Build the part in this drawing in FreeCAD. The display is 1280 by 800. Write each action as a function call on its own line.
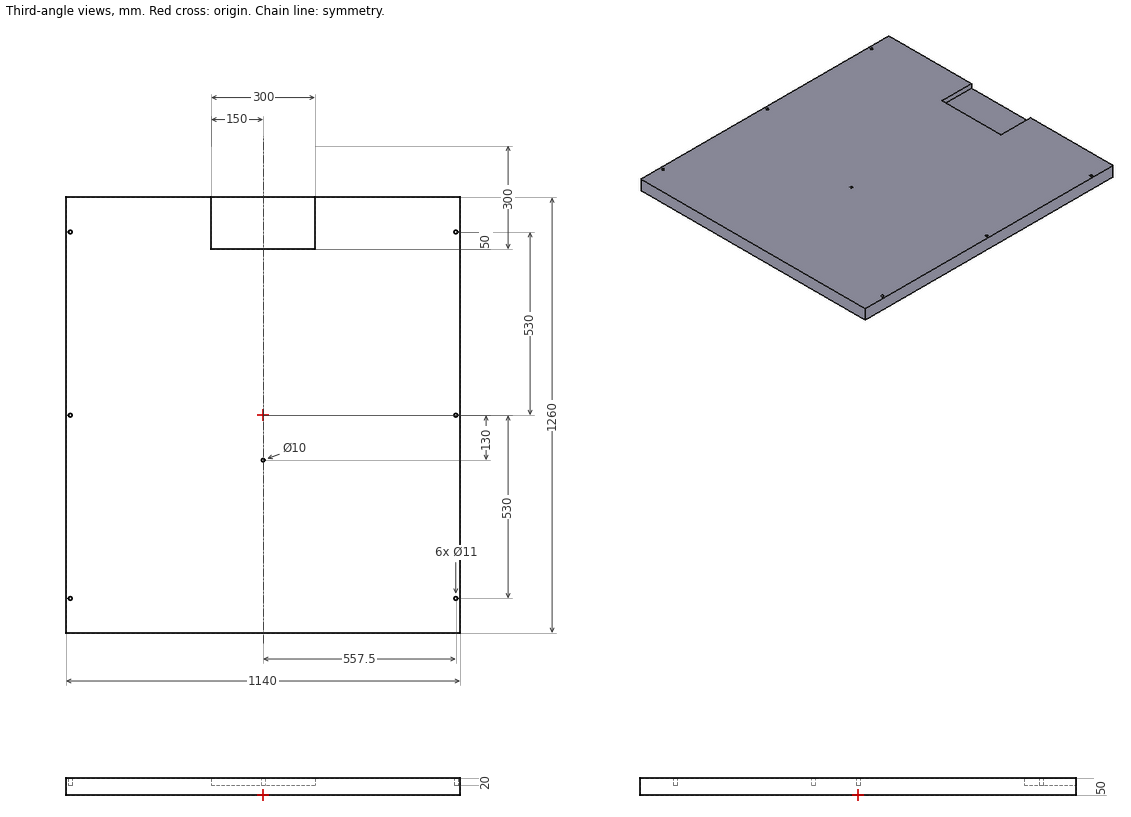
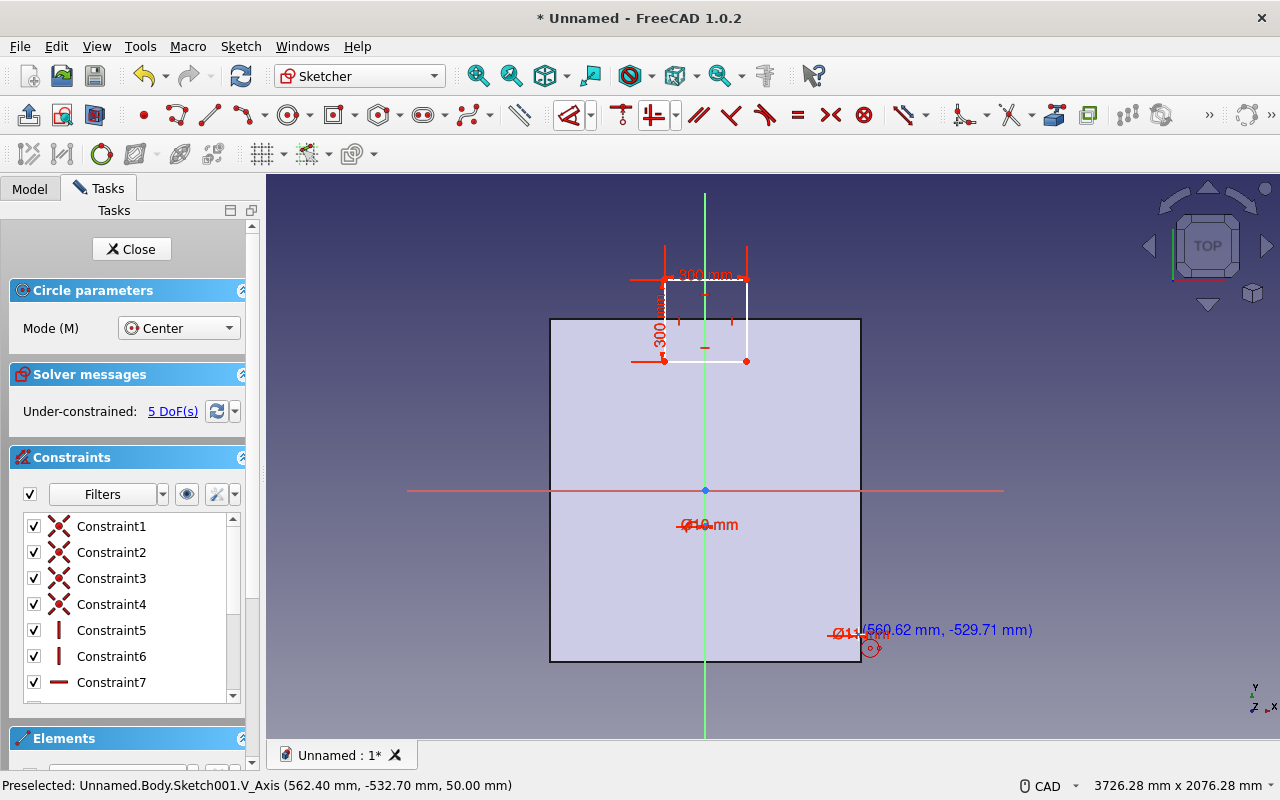
scroll(857, 491, up, 14)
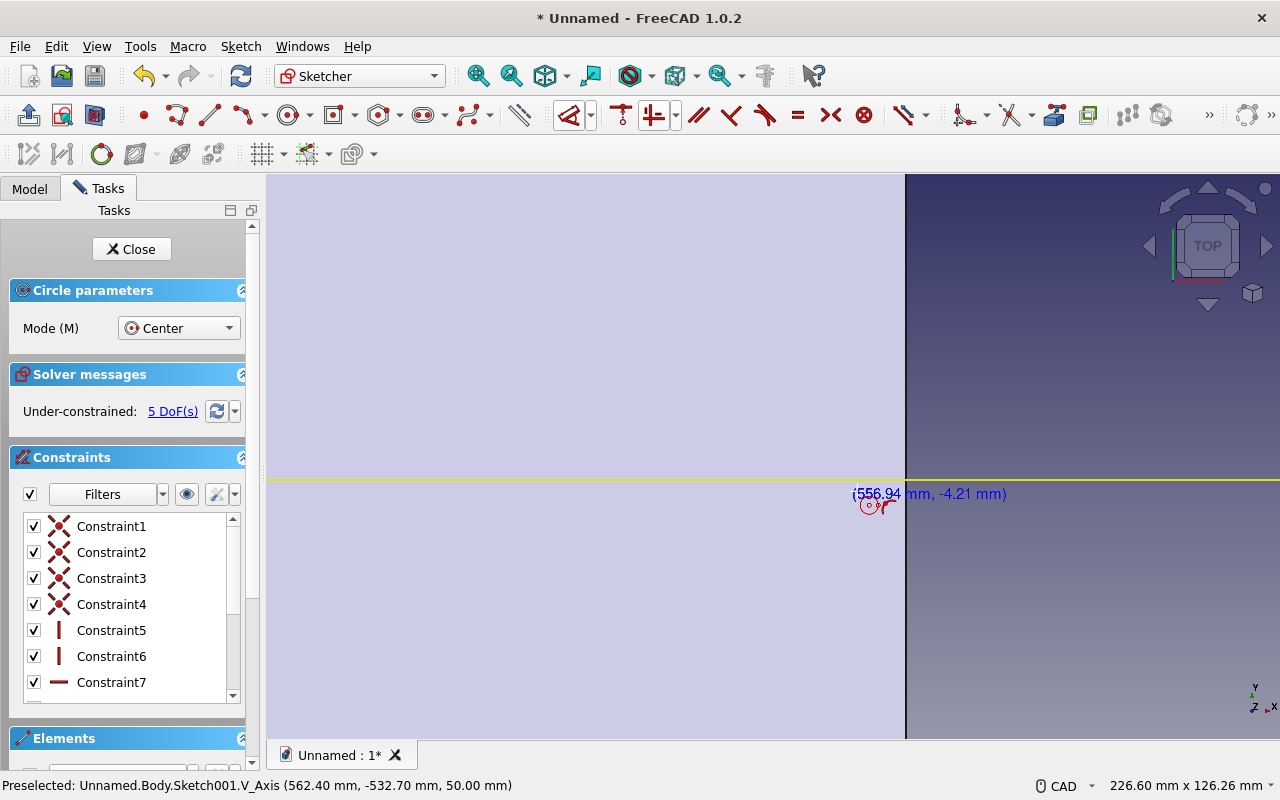
scroll(857, 490, down, 14)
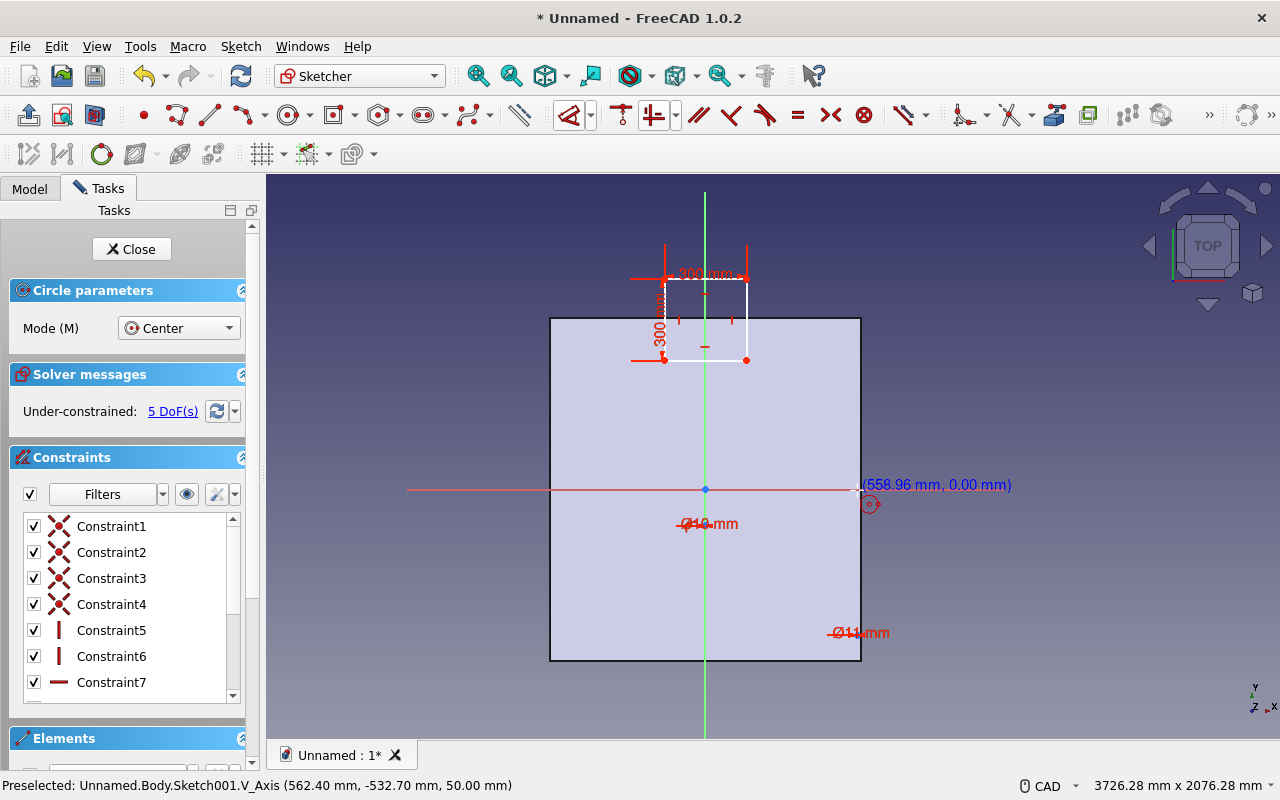
click(857, 490)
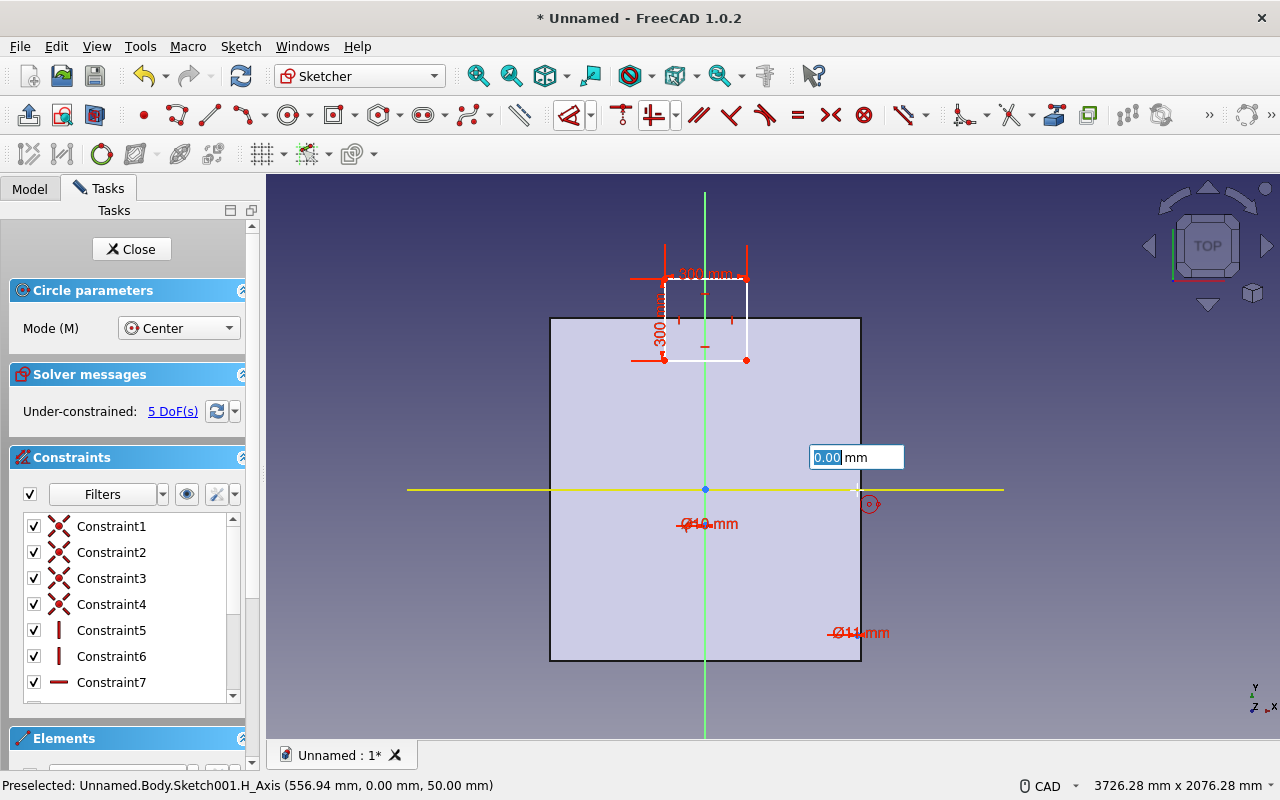
scroll(858, 489, up, 13)
move(846, 475)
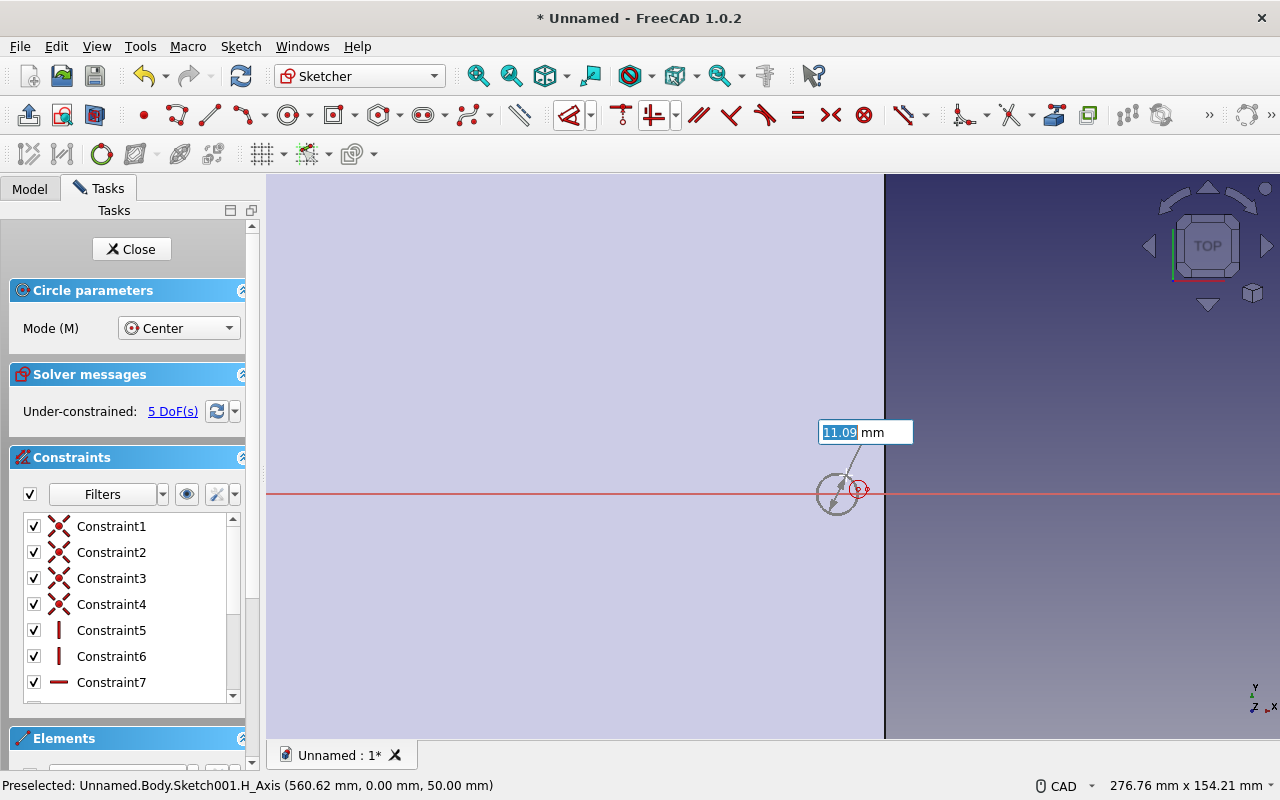
text(11)
key(Return)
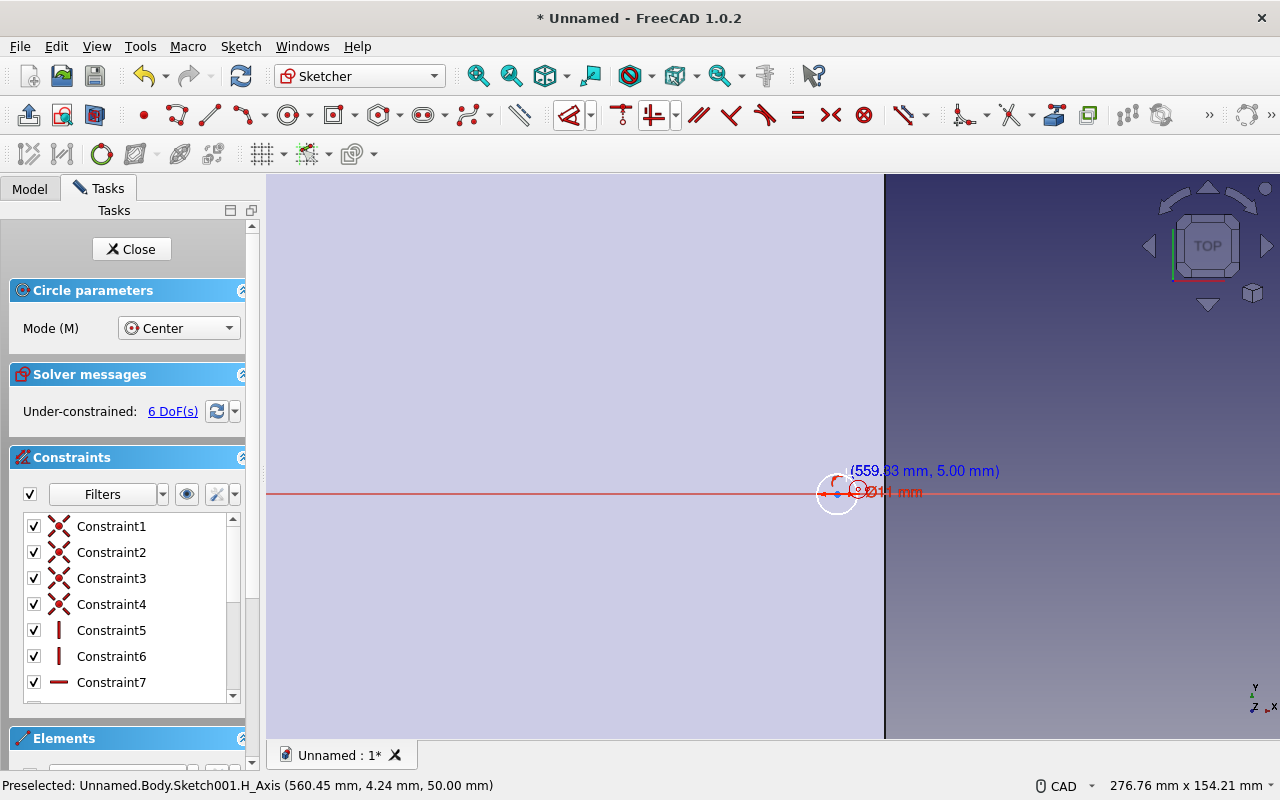
scroll(858, 489, down, 13)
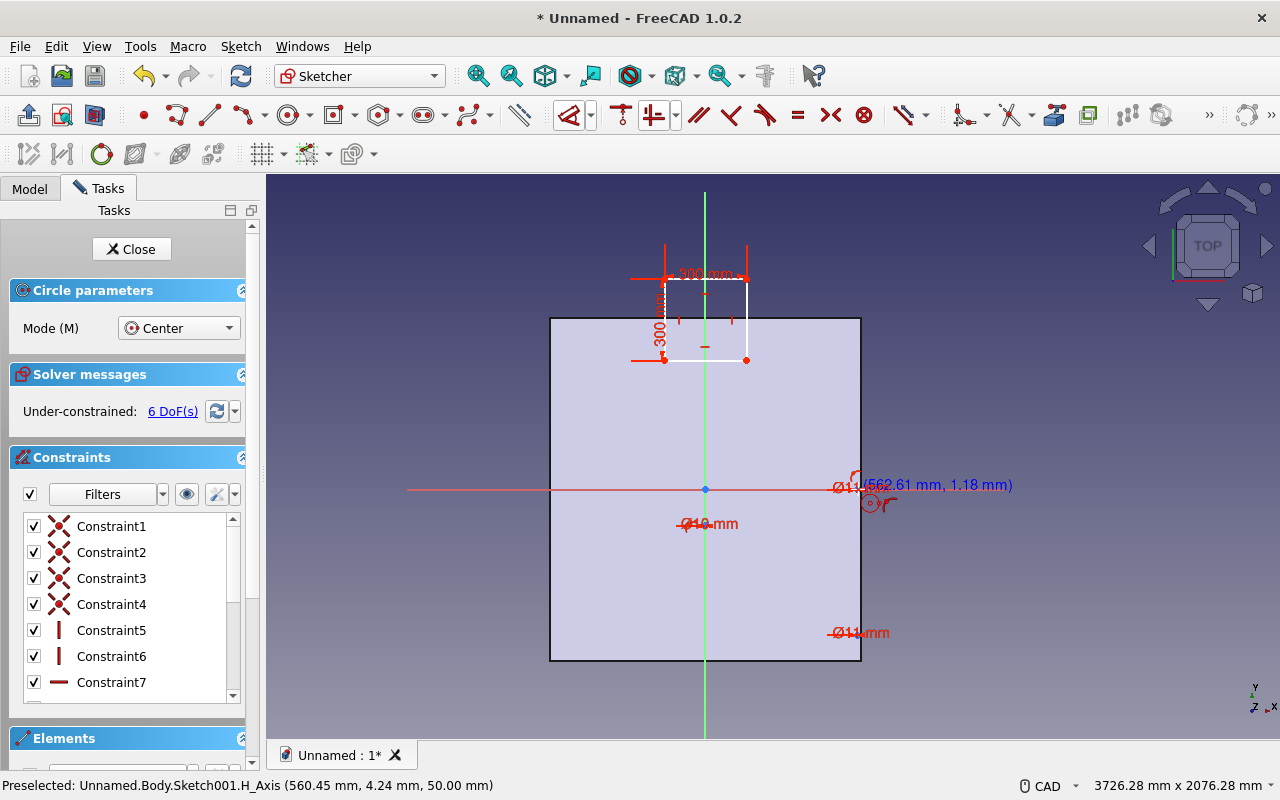
scroll(857, 346, up, 14)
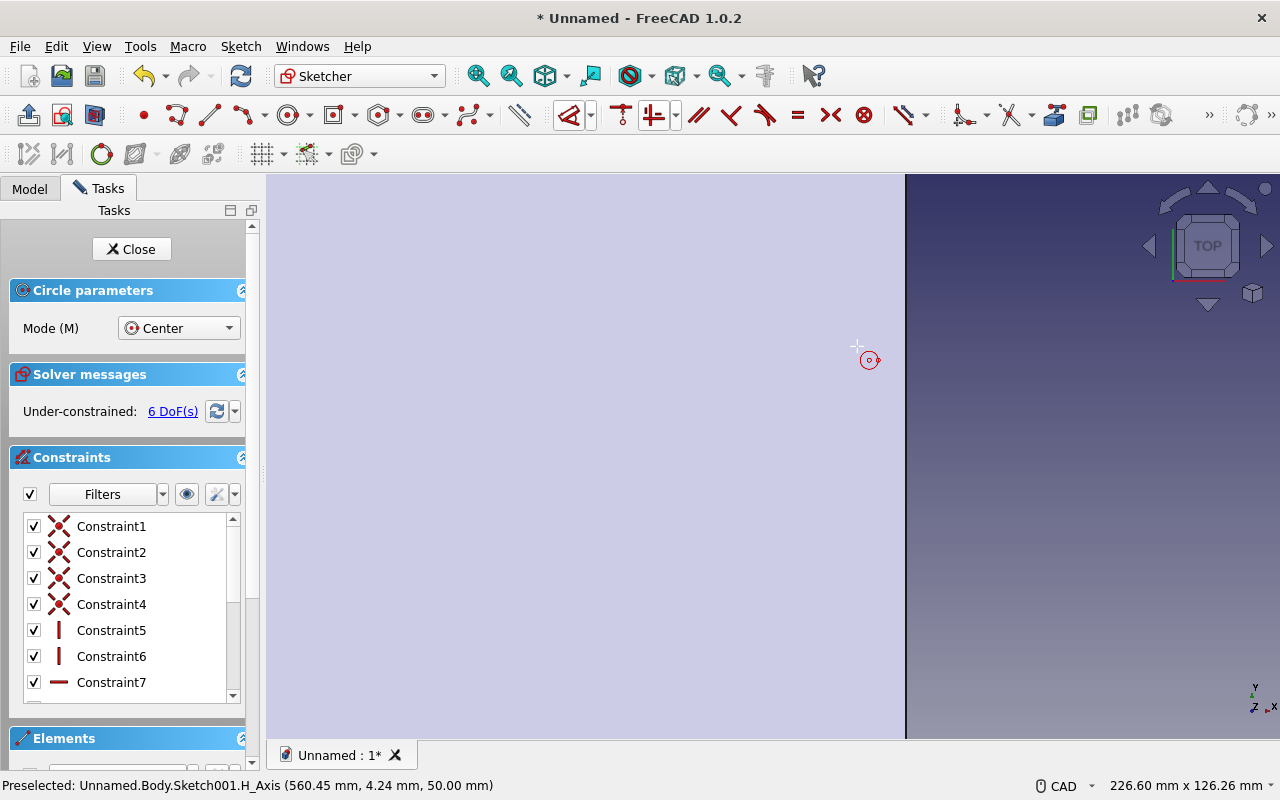
scroll(857, 346, down, 14)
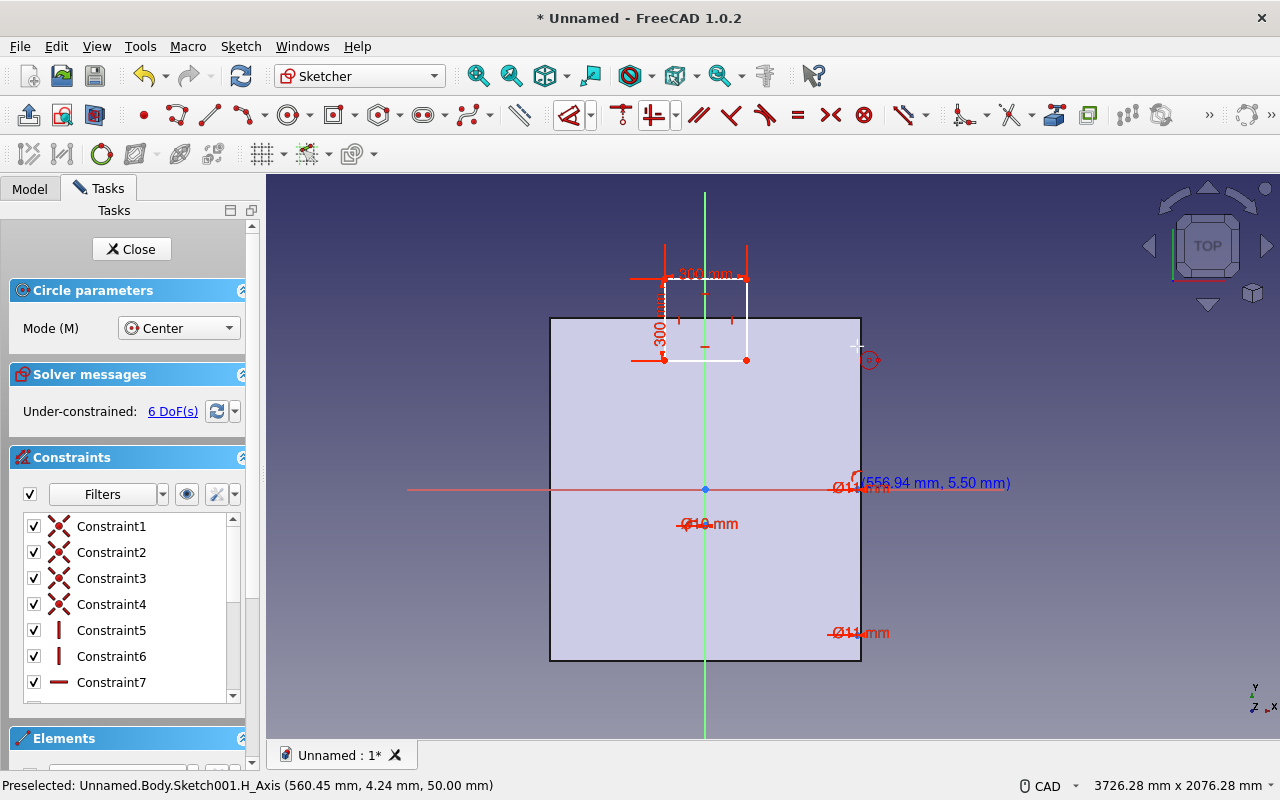
click(857, 346)
move(858, 345)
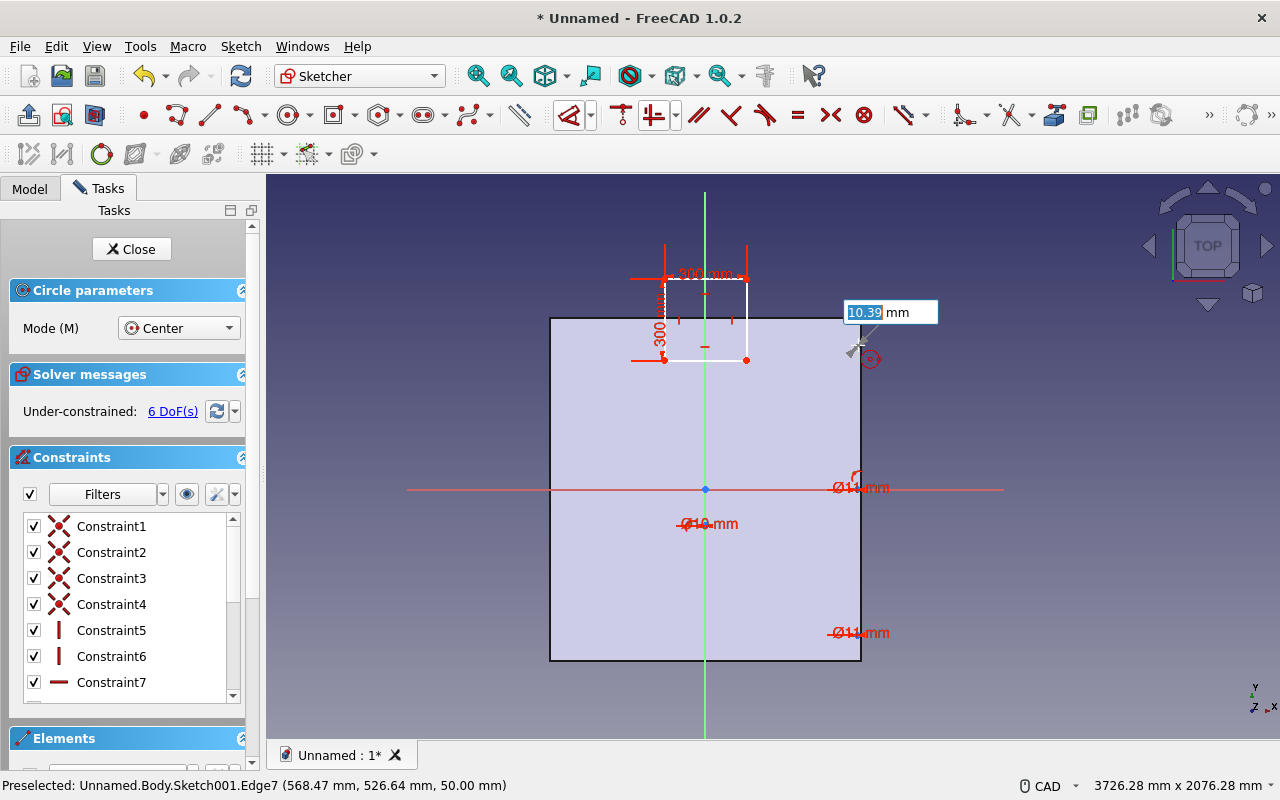
text(11)
key(Return)